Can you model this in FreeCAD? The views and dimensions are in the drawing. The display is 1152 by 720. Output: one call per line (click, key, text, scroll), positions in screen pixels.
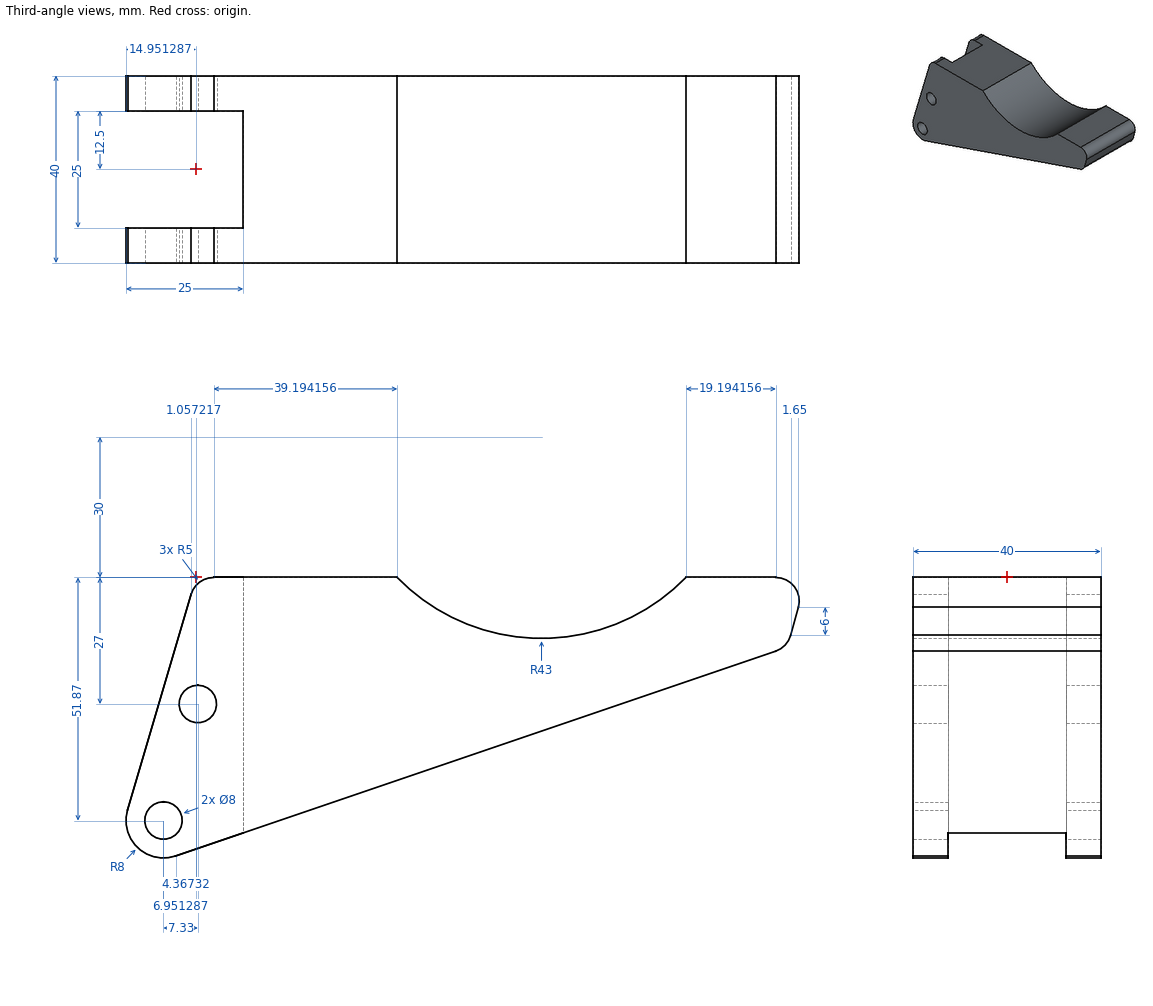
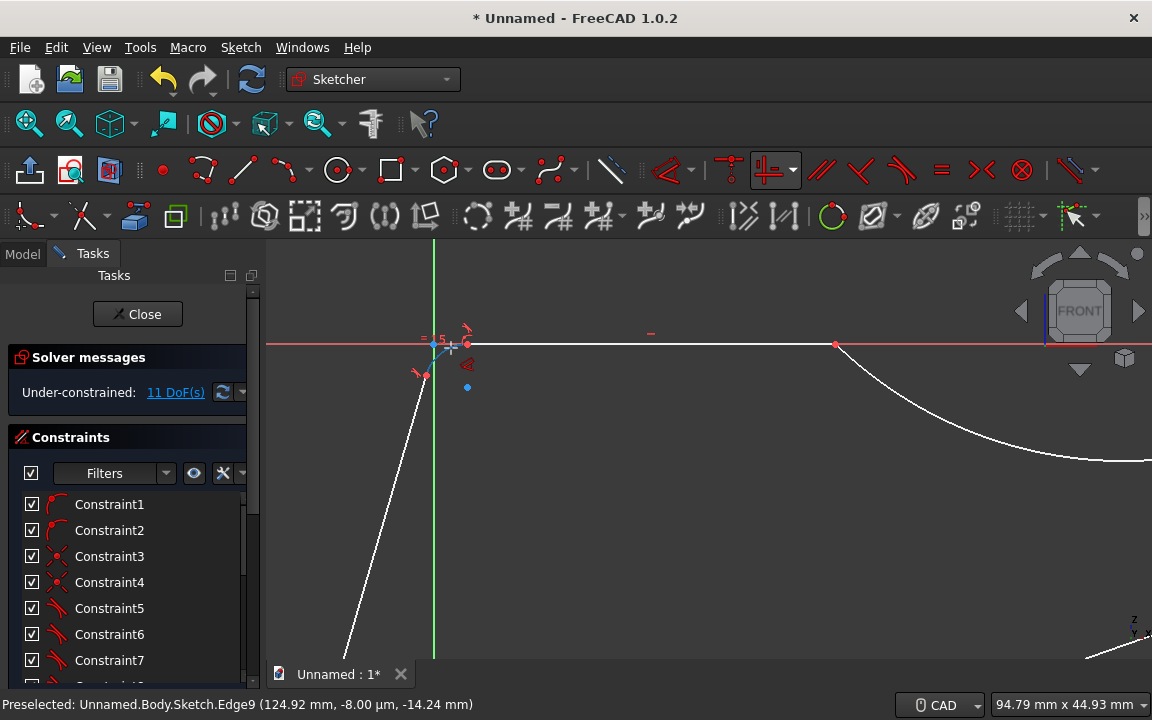
click(451, 347)
click(476, 312)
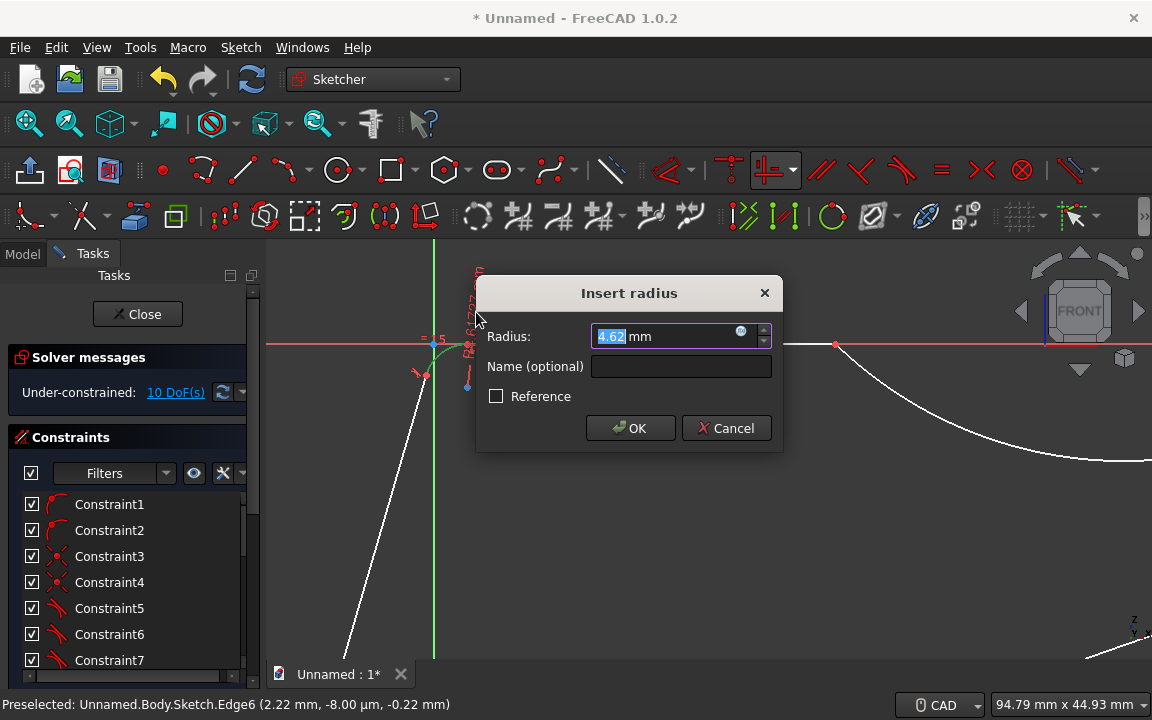
text(5)
key(Return)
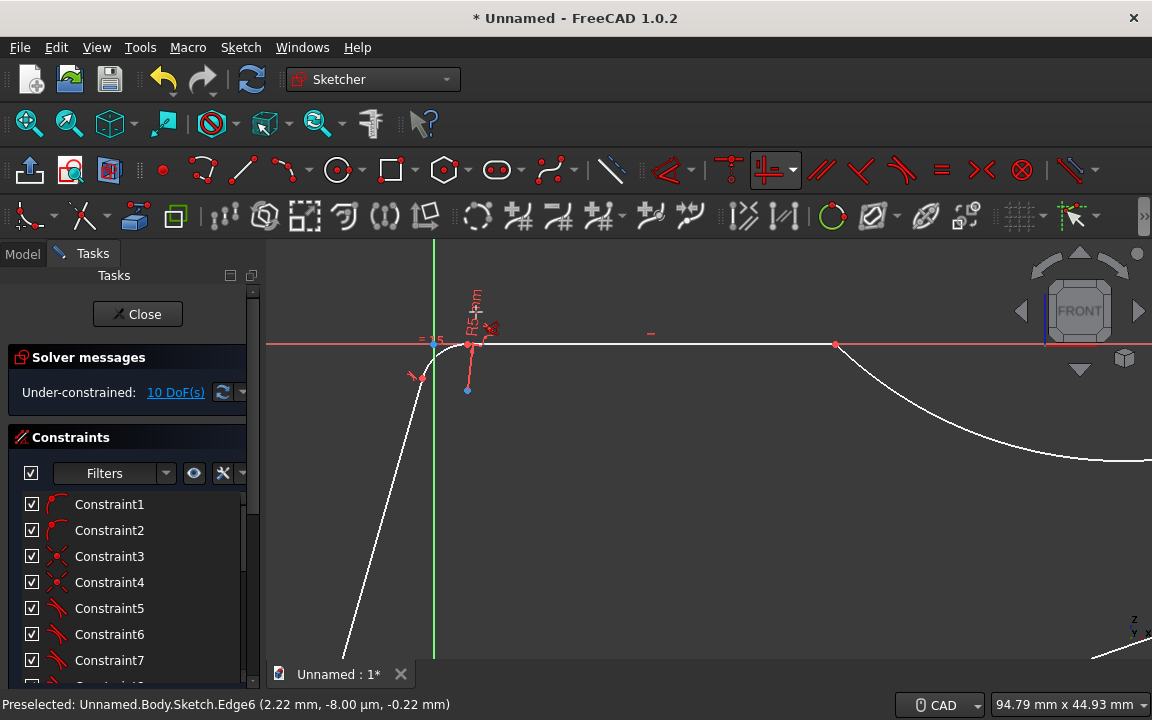
click(939, 418)
click(925, 447)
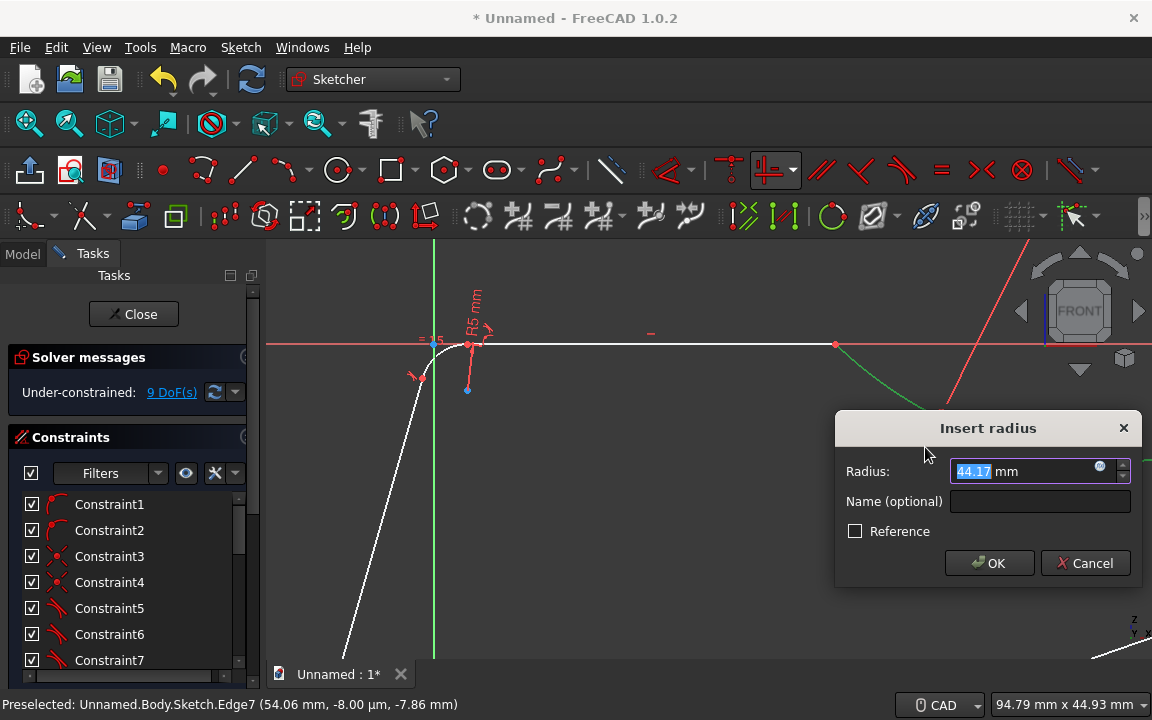
text(43)
key(Return)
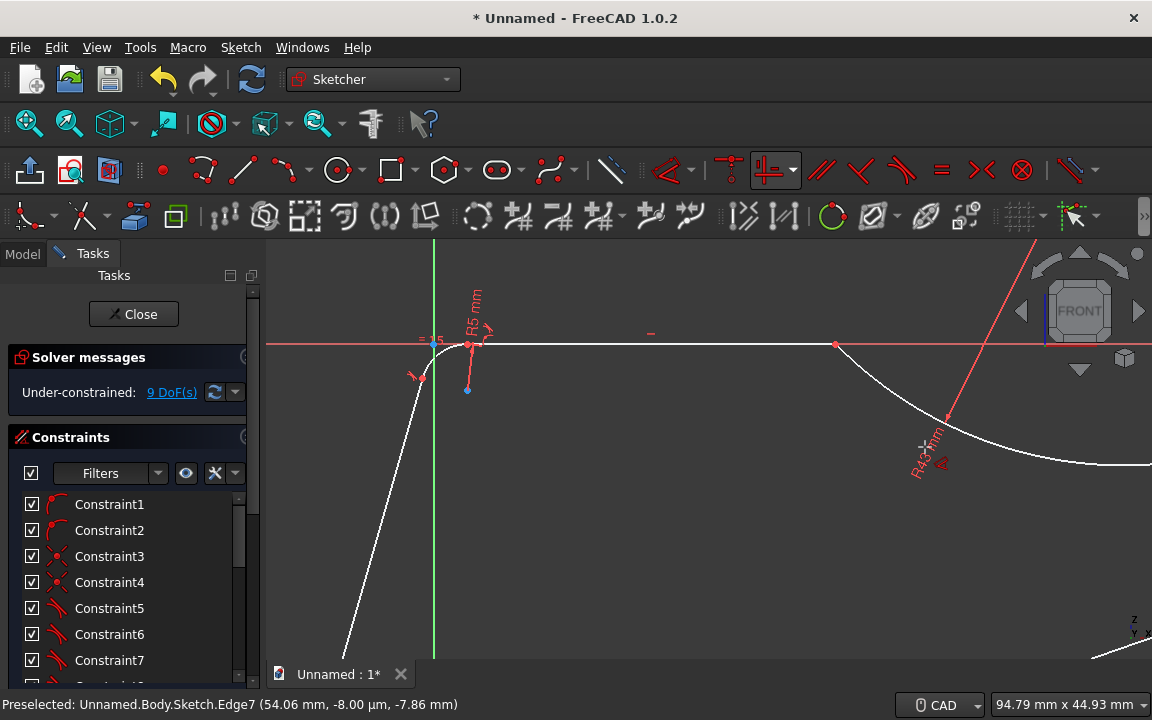
scroll(451, 348, down, 5)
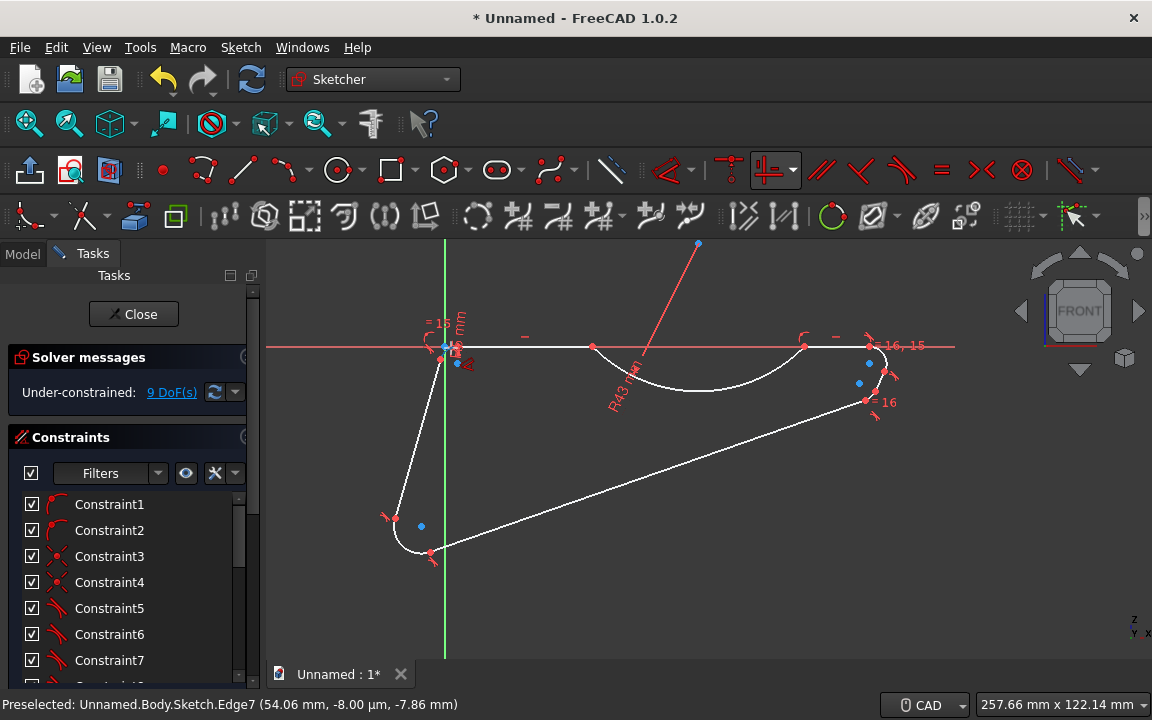
scroll(396, 536, up, 2)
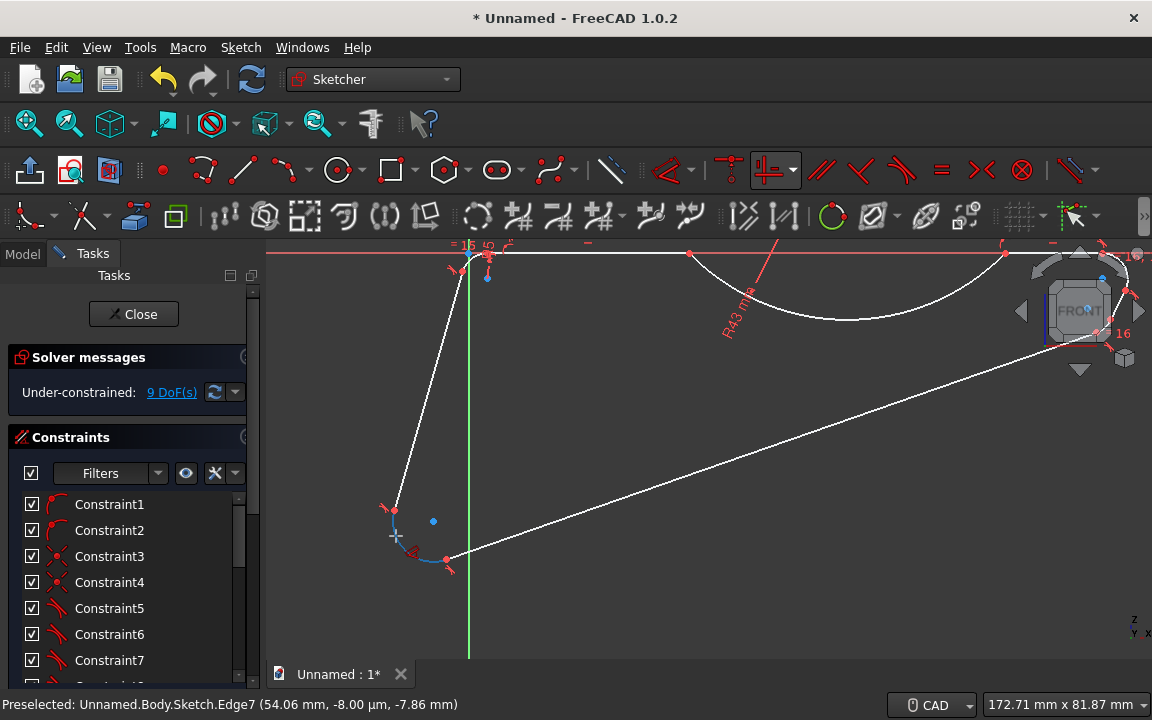
click(396, 536)
click(366, 548)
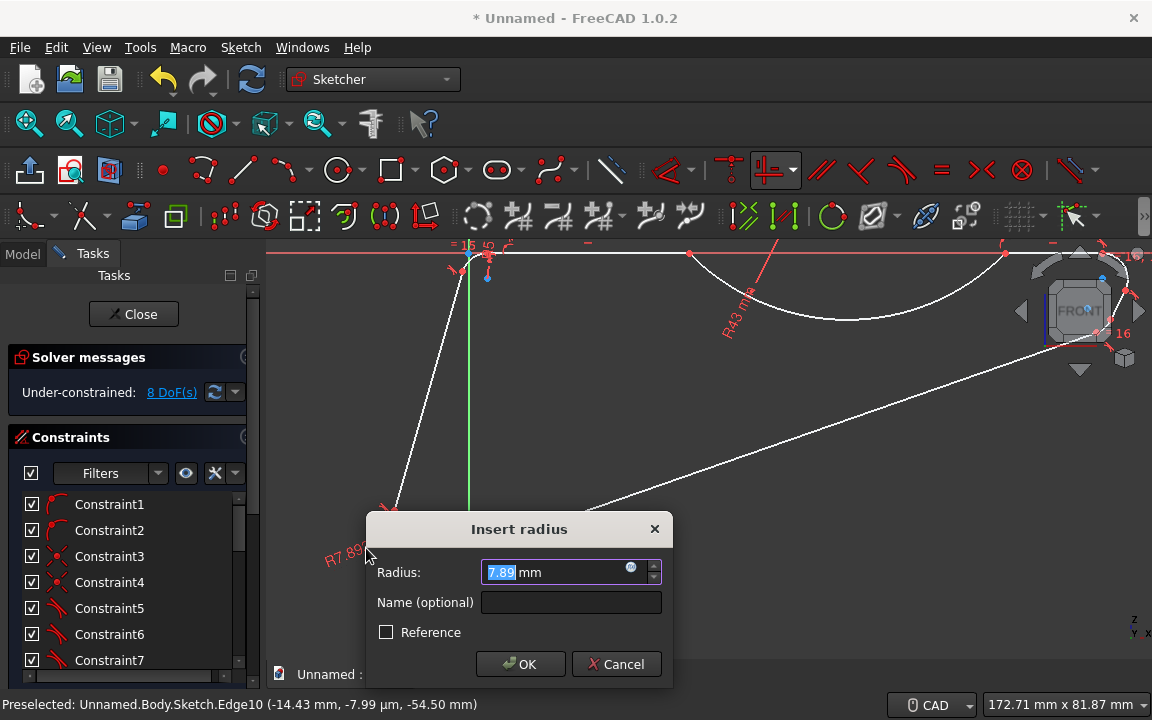
text(8)
key(Return)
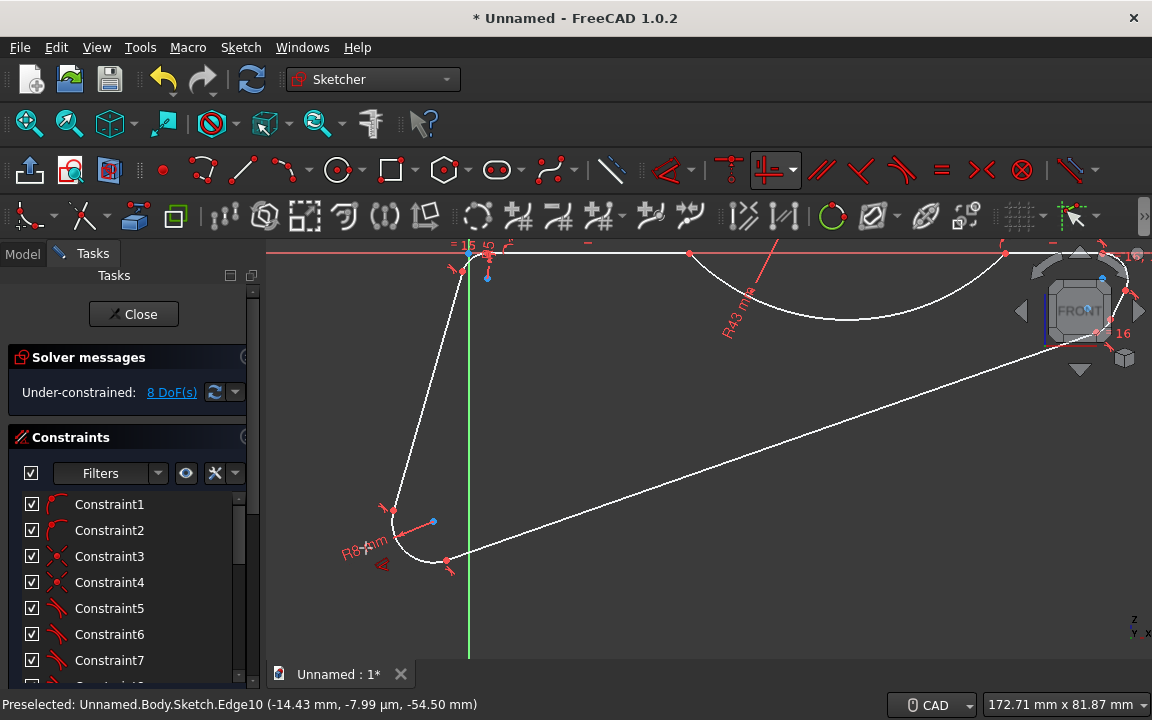
scroll(395, 537, down, 2)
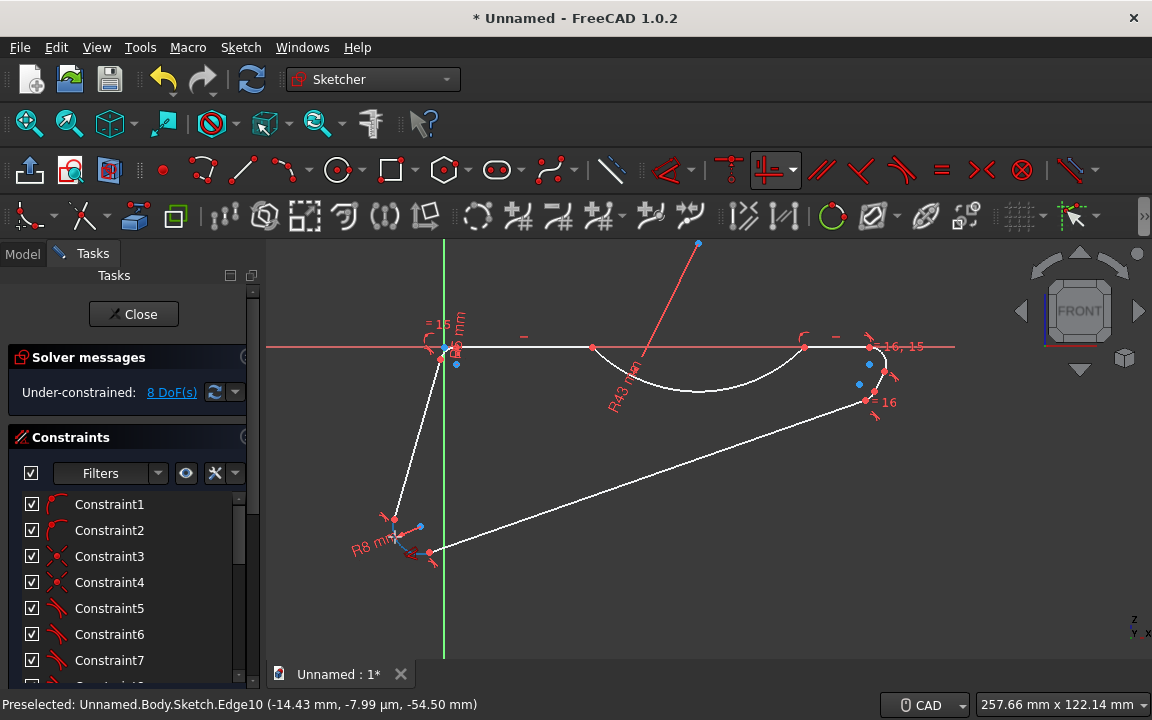
scroll(882, 378, up, 4)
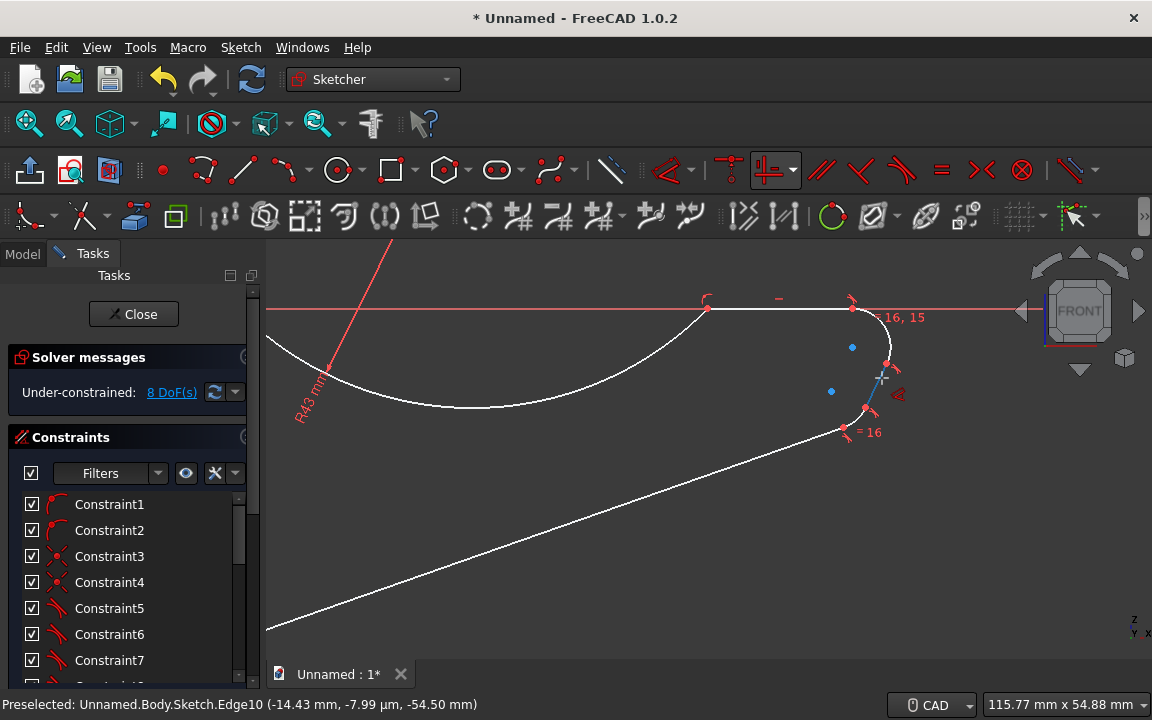
click(880, 377)
click(921, 386)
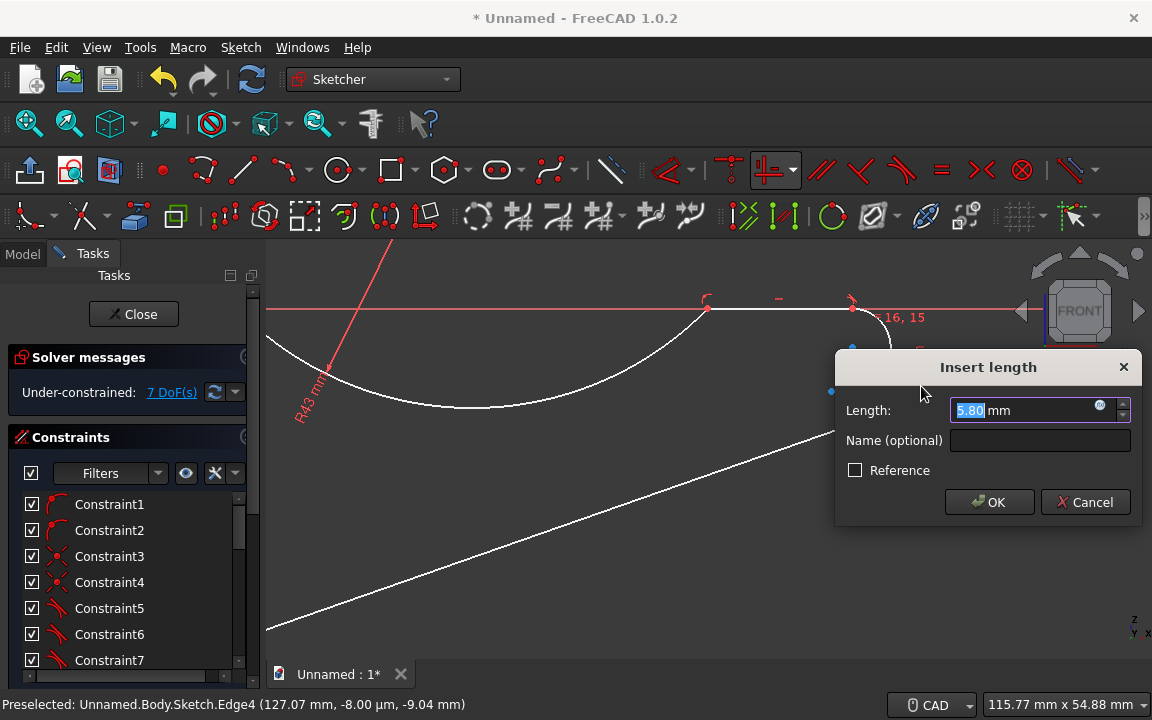
text(6)
key(Return)